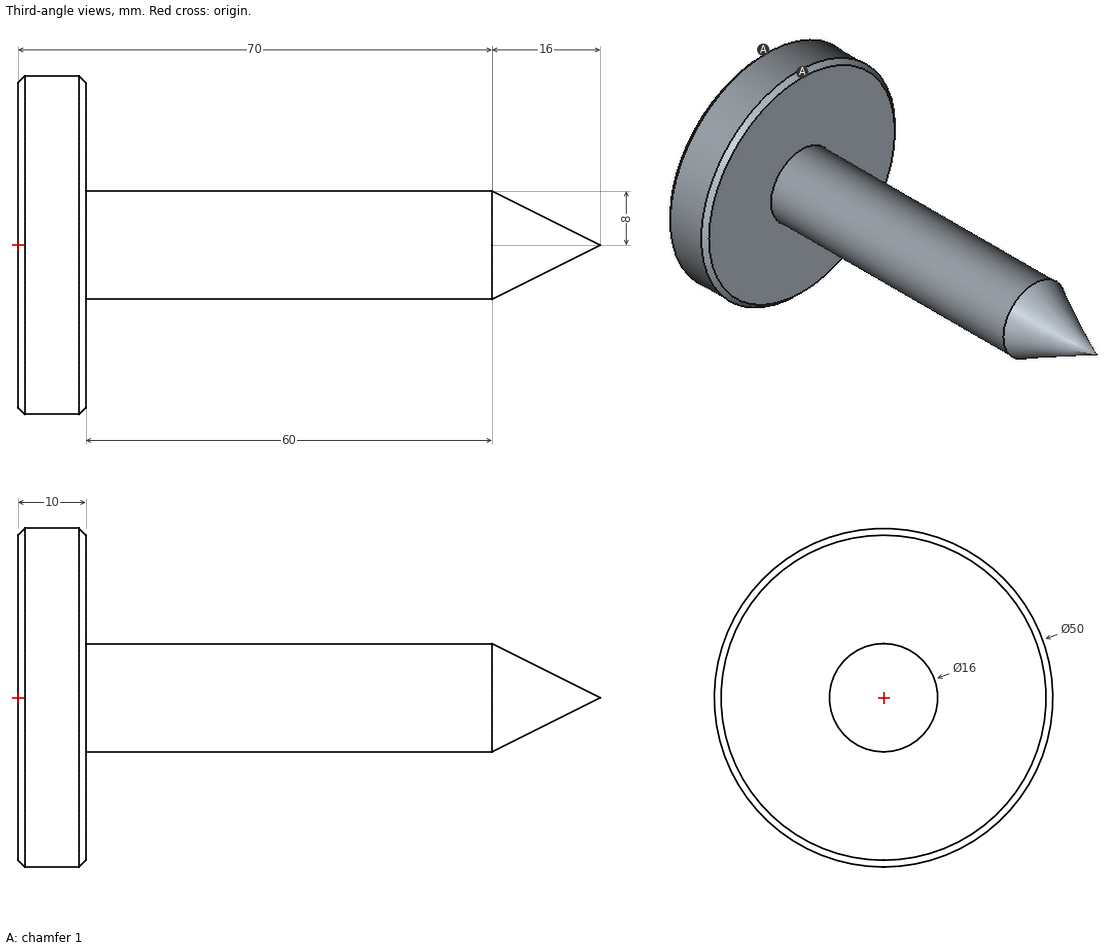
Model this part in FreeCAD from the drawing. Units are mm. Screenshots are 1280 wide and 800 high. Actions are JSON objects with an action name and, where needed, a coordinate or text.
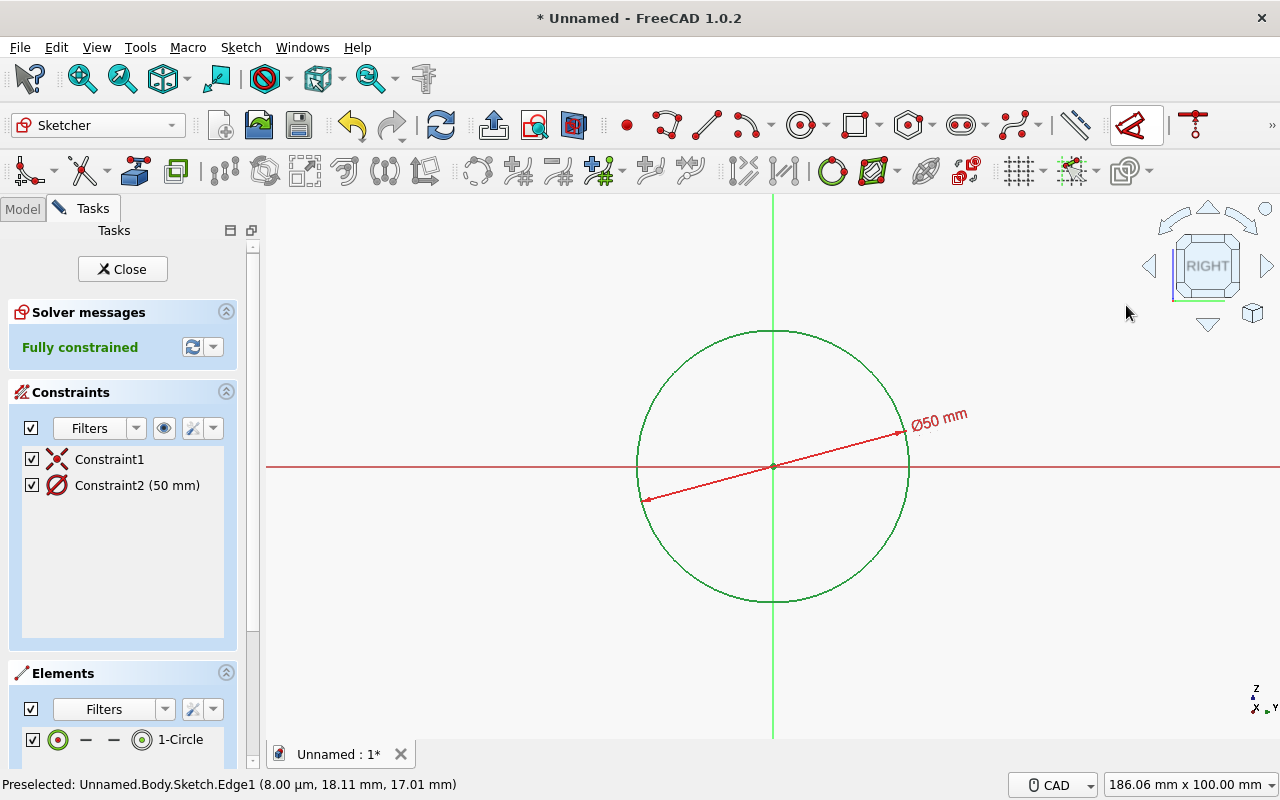
{"action": "left_click", "coordinate": [123, 269]}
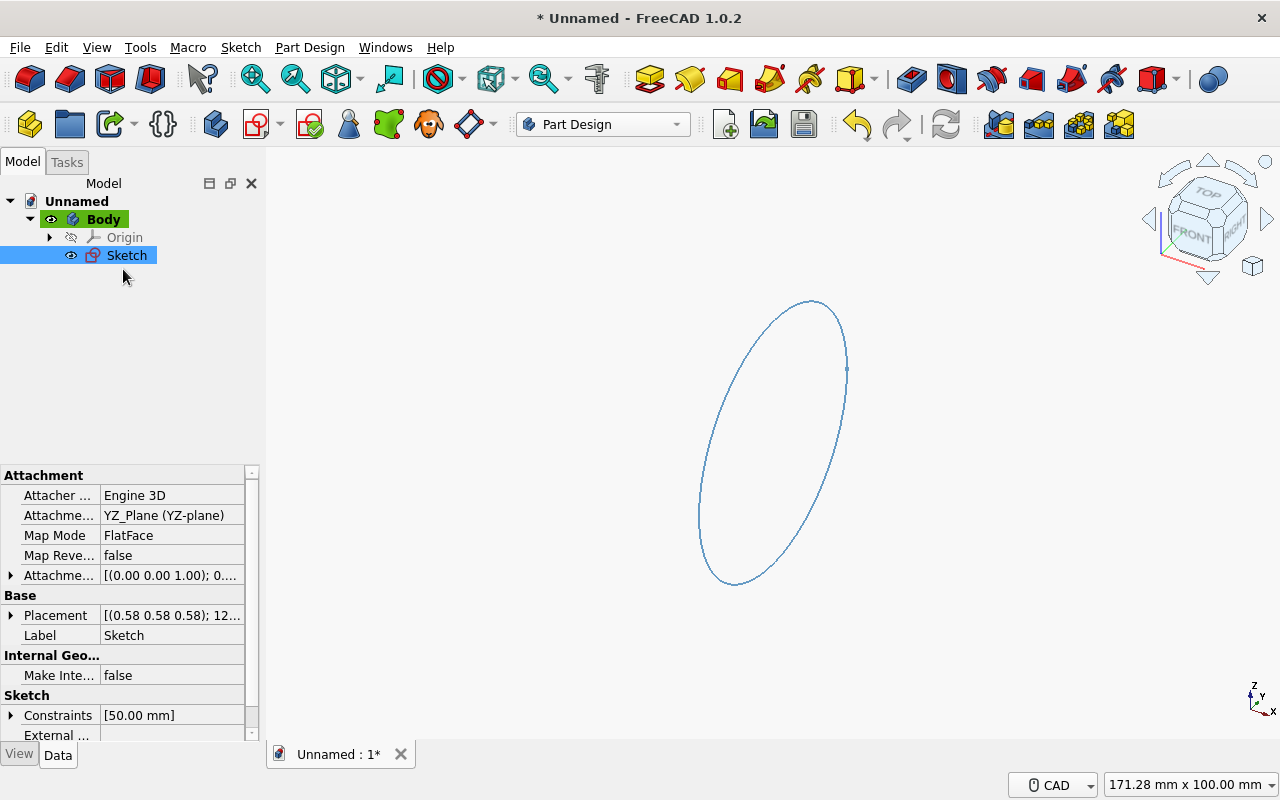
{"action": "left_click", "coordinate": [650, 80]}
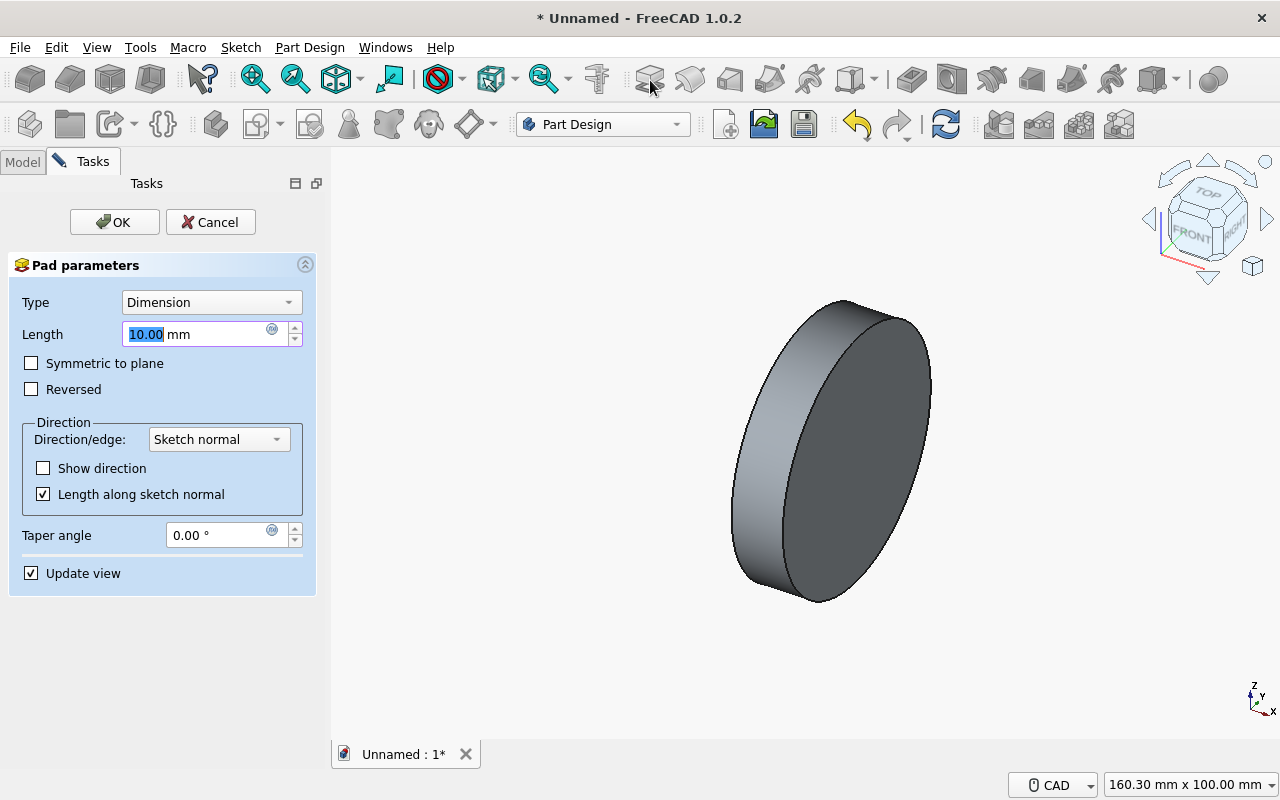
{"action": "type", "text": "10"}
{"action": "key", "text": "Tab"}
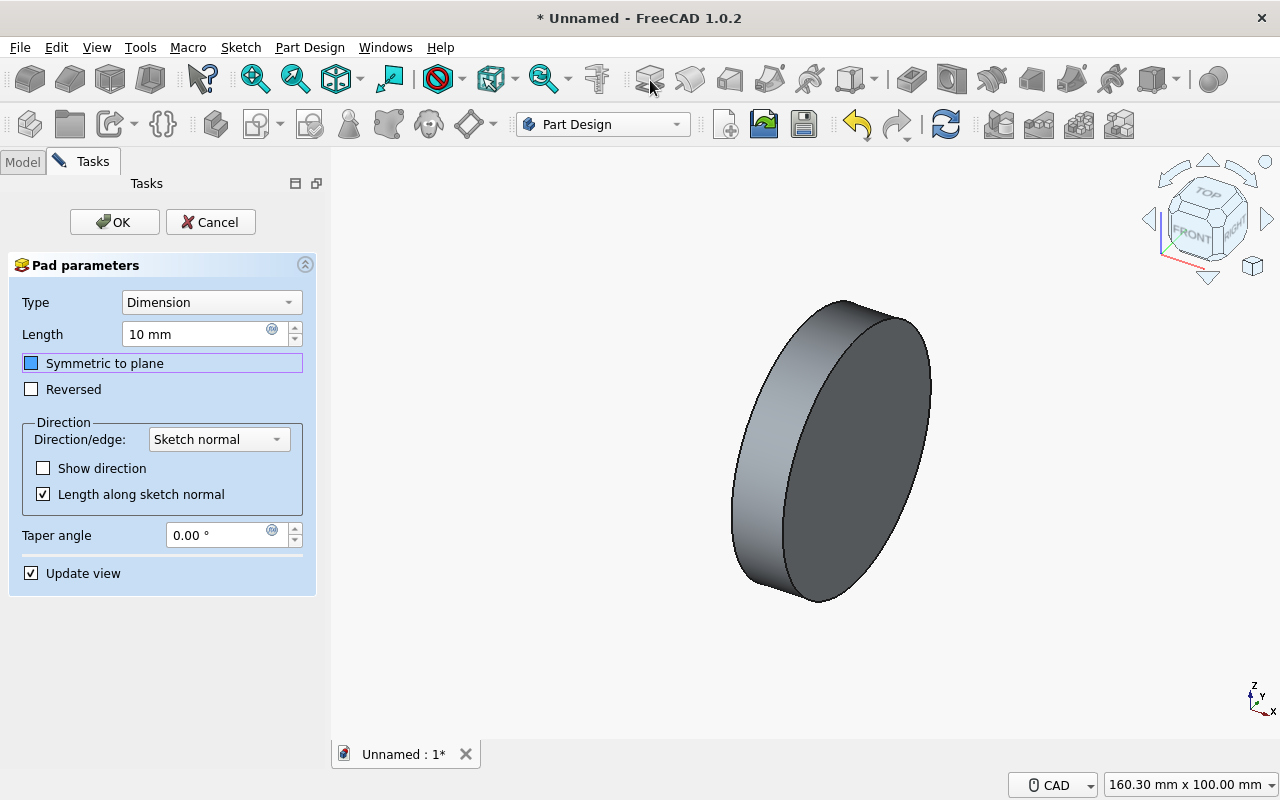
{"action": "left_click", "coordinate": [115, 222]}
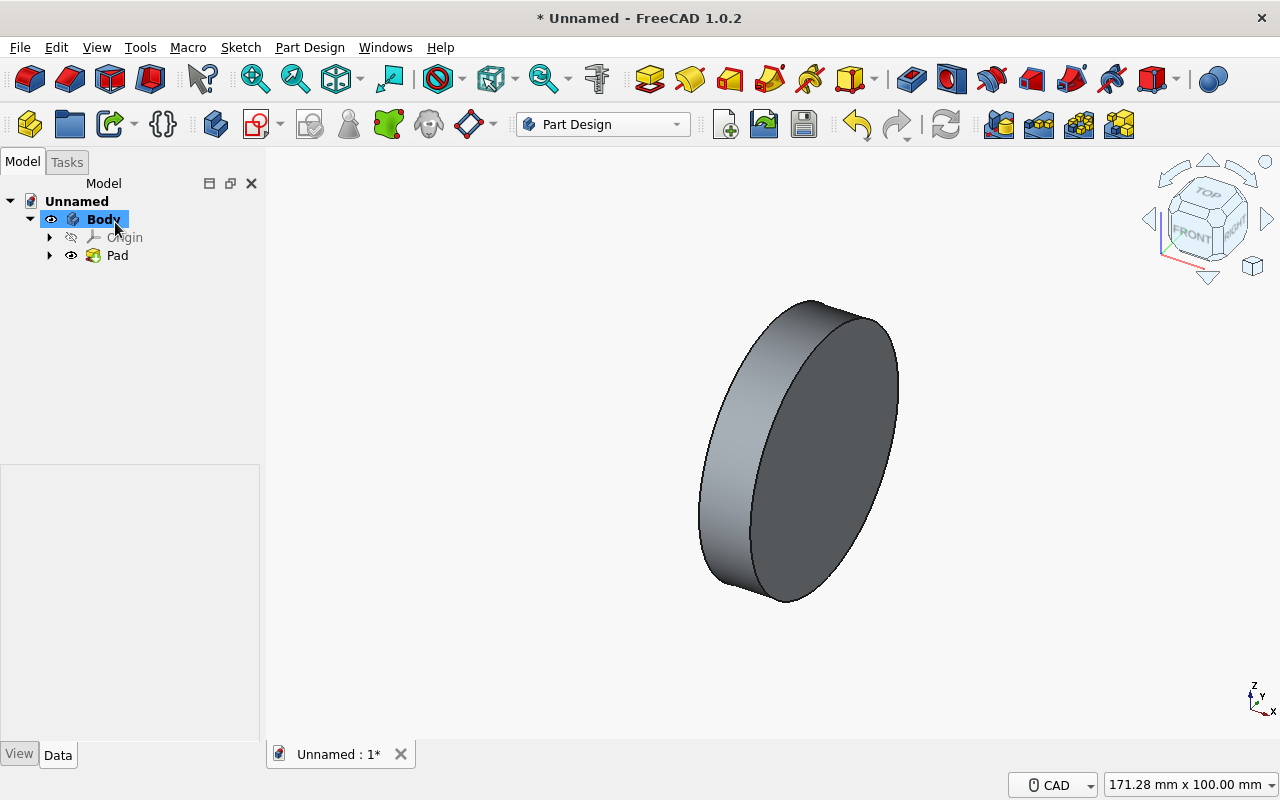
{"action": "left_click", "coordinate": [824, 459]}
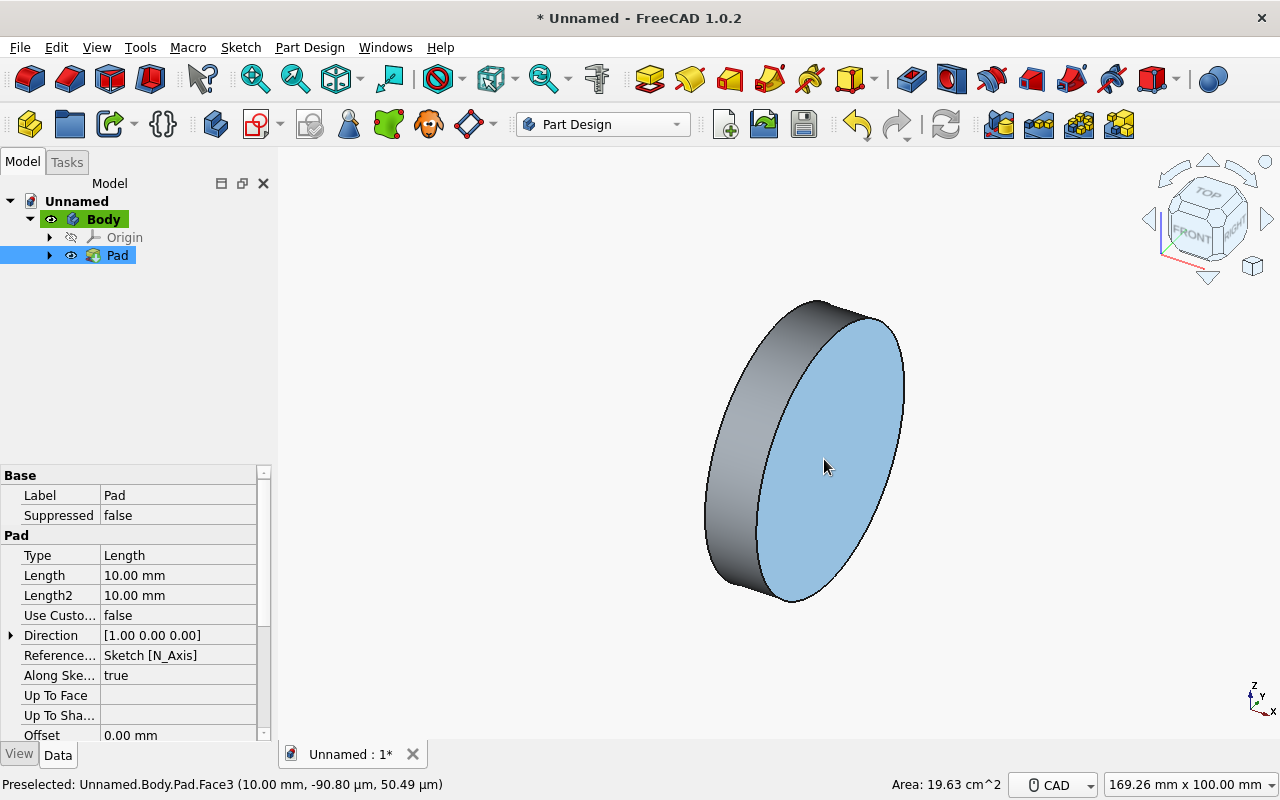
{"action": "left_click", "coordinate": [256, 124]}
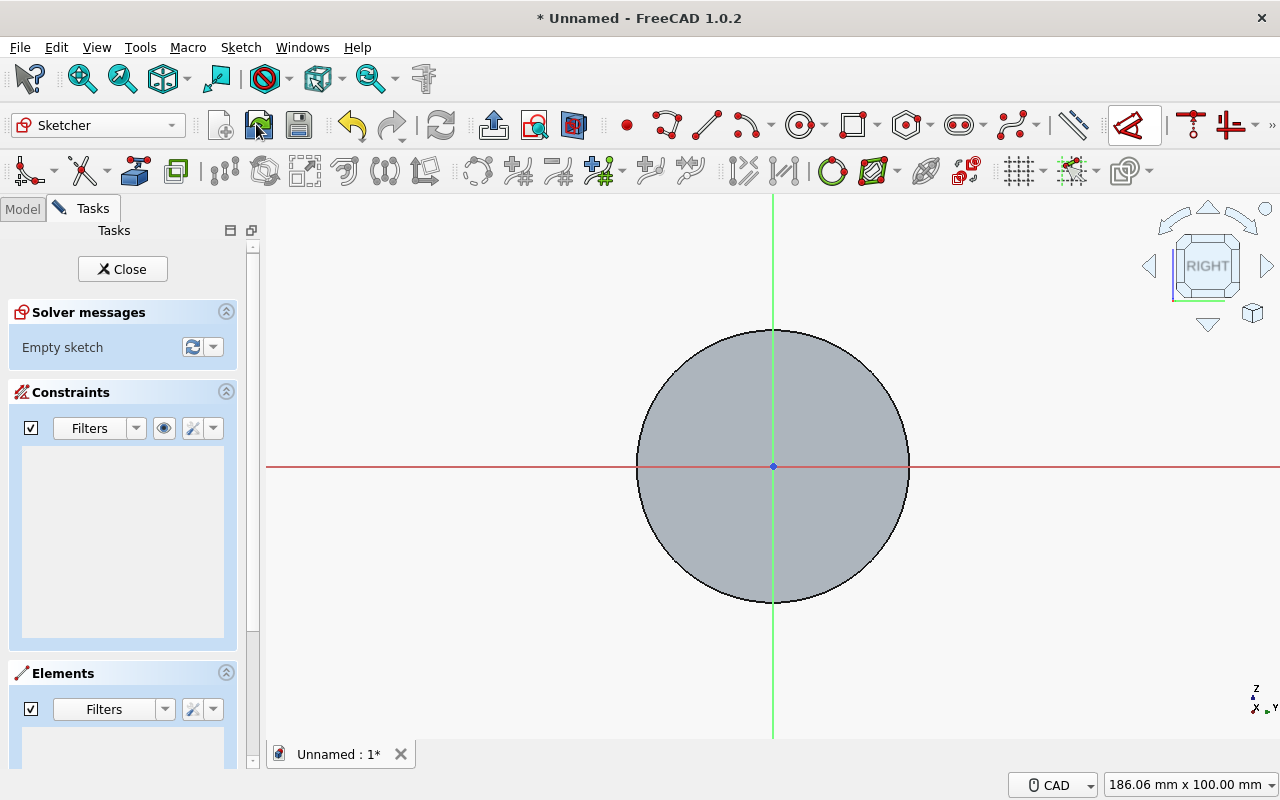
{"action": "scroll", "coordinate": [795, 466], "scroll_direction": "up", "scroll_amount": 7}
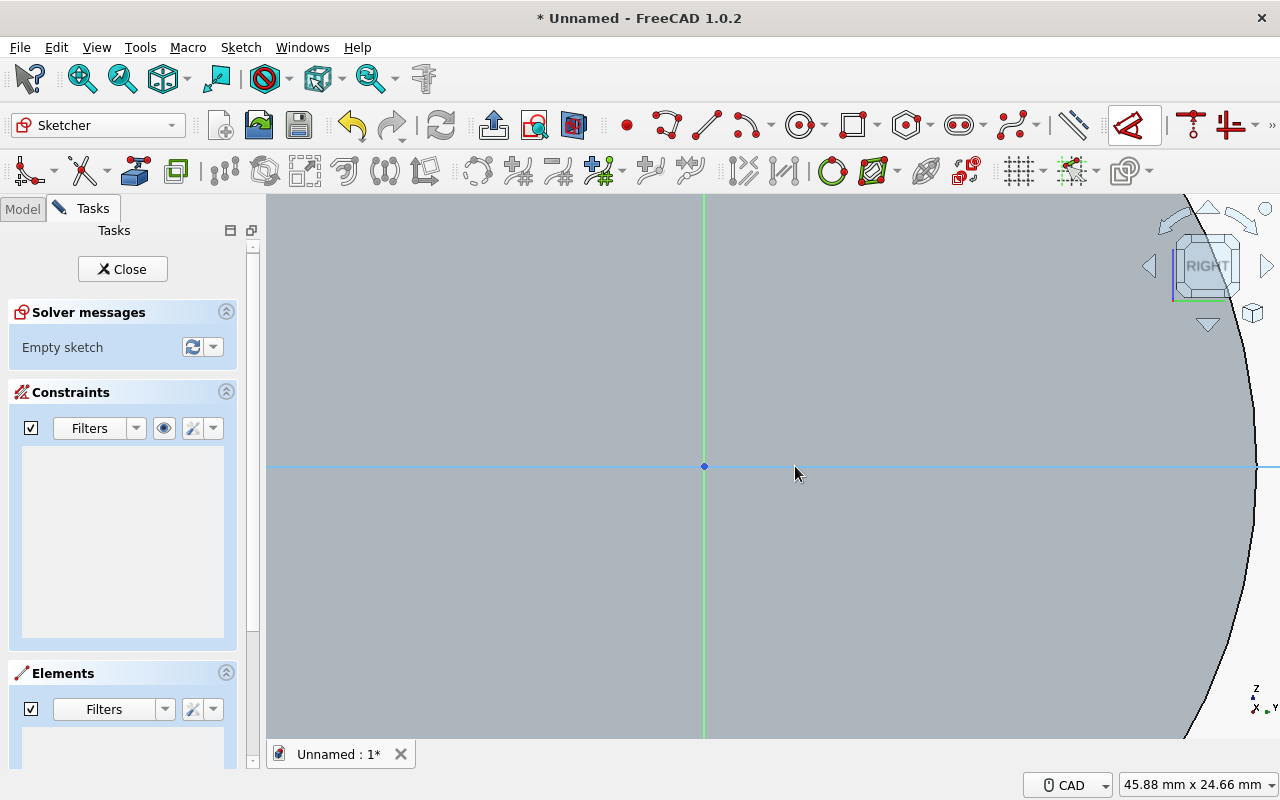
{"action": "key", "text": "g c"}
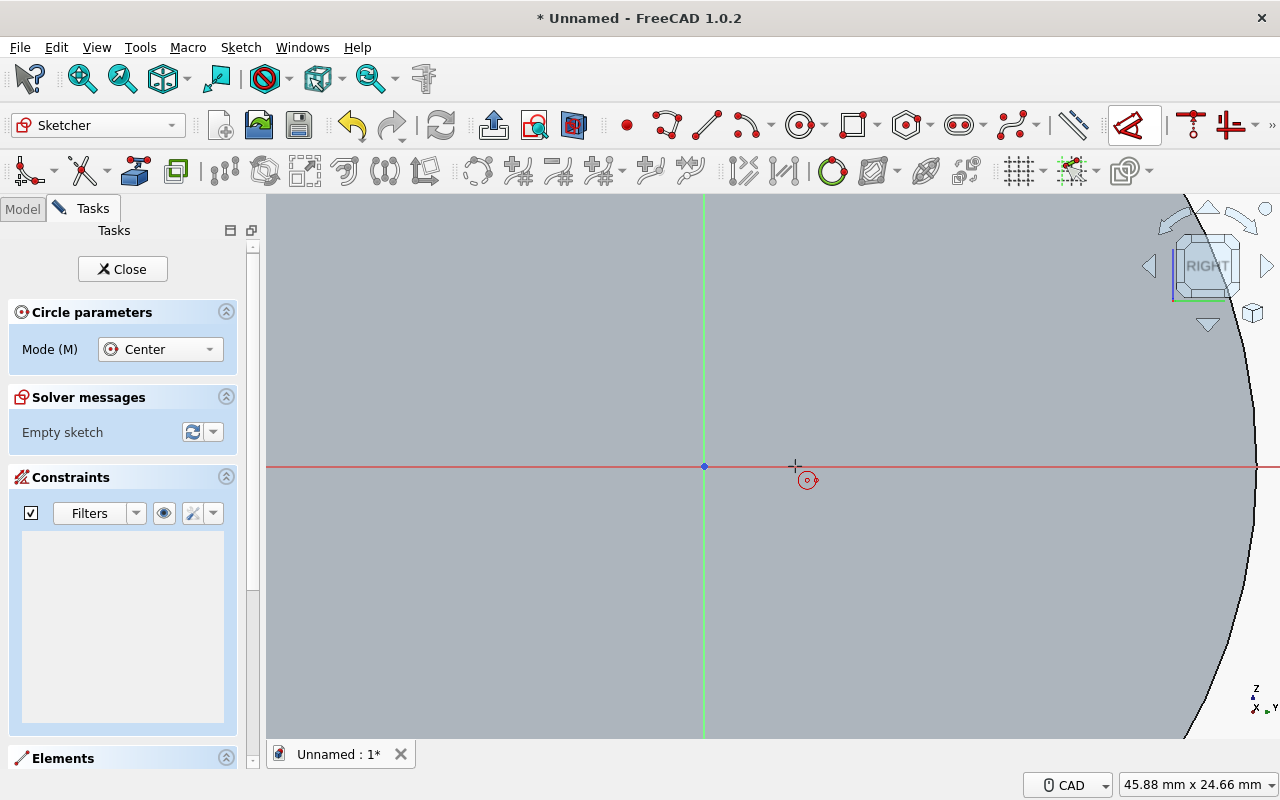
{"action": "left_click", "coordinate": [704, 466]}
{"action": "left_click", "coordinate": [829, 341]}
{"action": "key", "text": "Escape"}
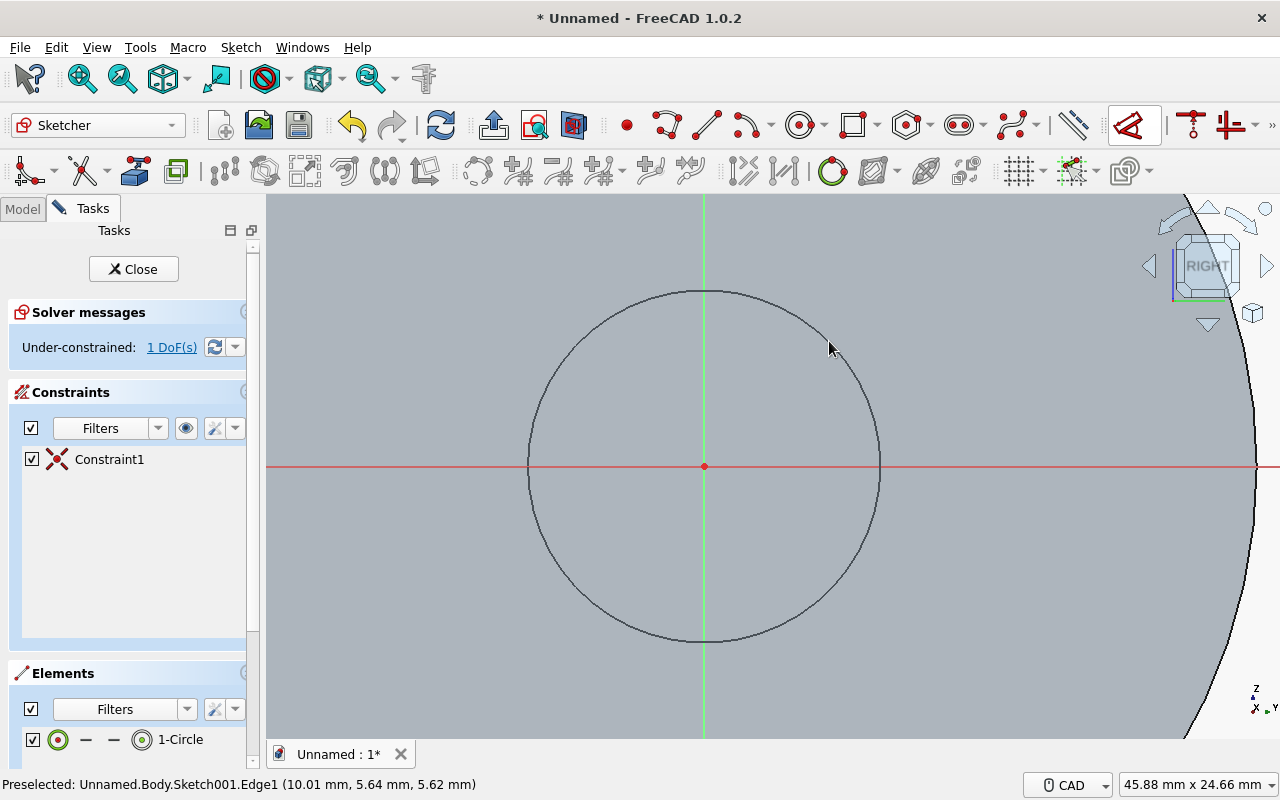
{"action": "left_click", "coordinate": [828, 341]}